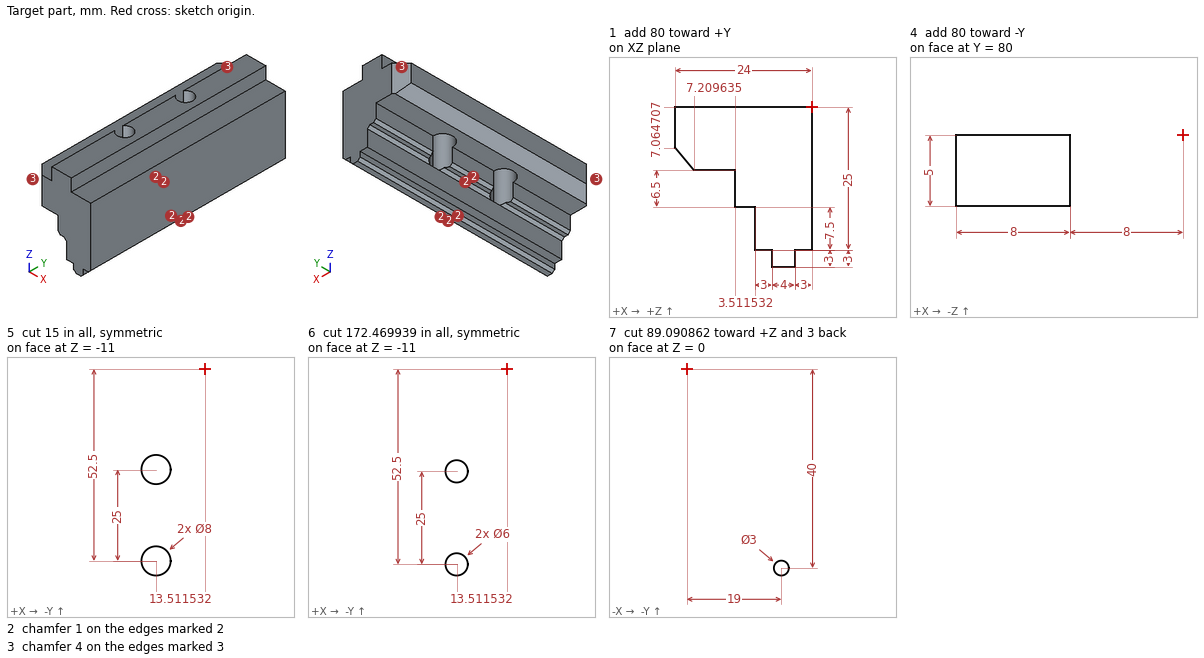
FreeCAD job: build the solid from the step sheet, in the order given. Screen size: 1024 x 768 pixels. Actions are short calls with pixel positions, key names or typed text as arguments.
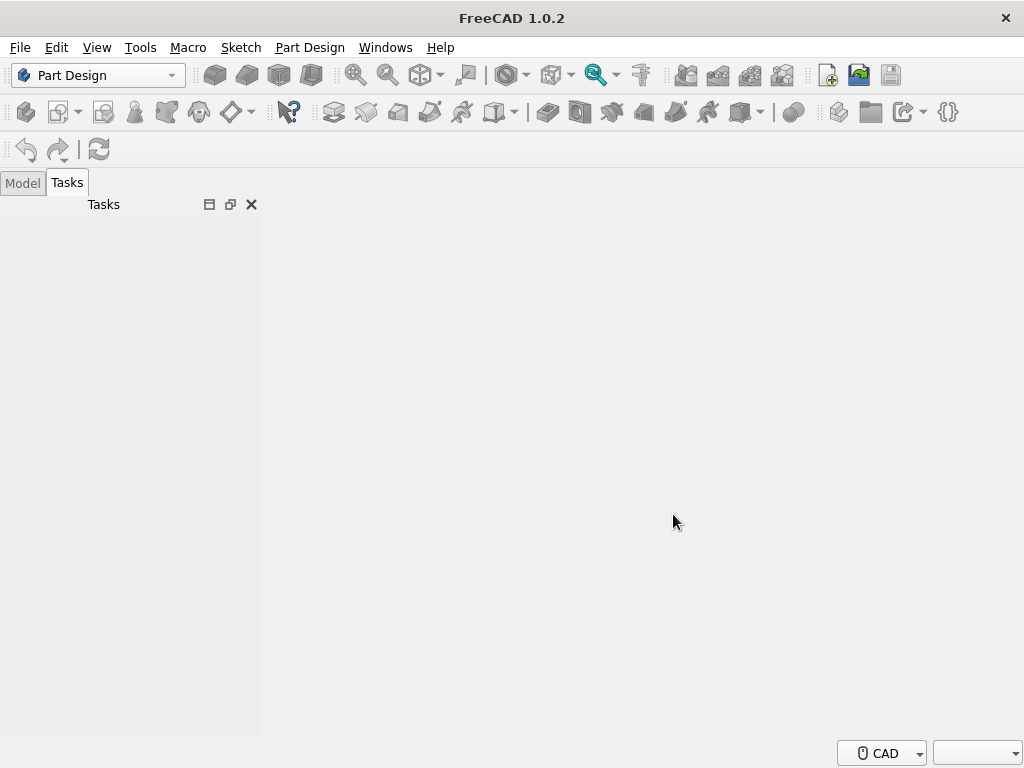
key(ctrl+n)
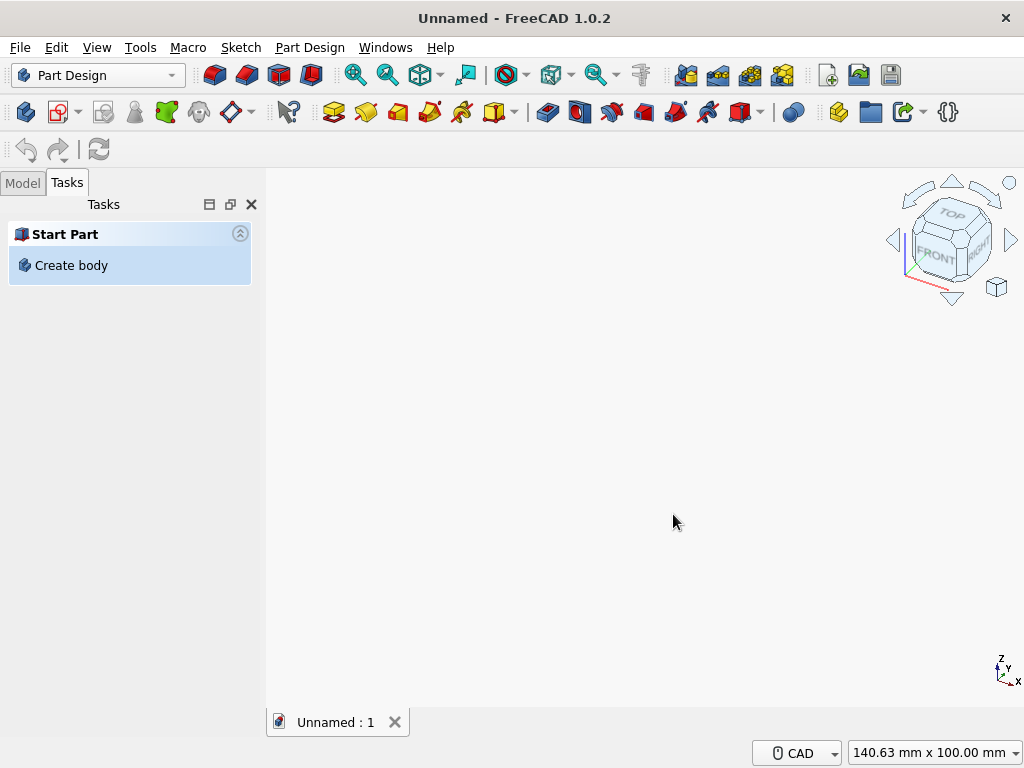
click(58, 112)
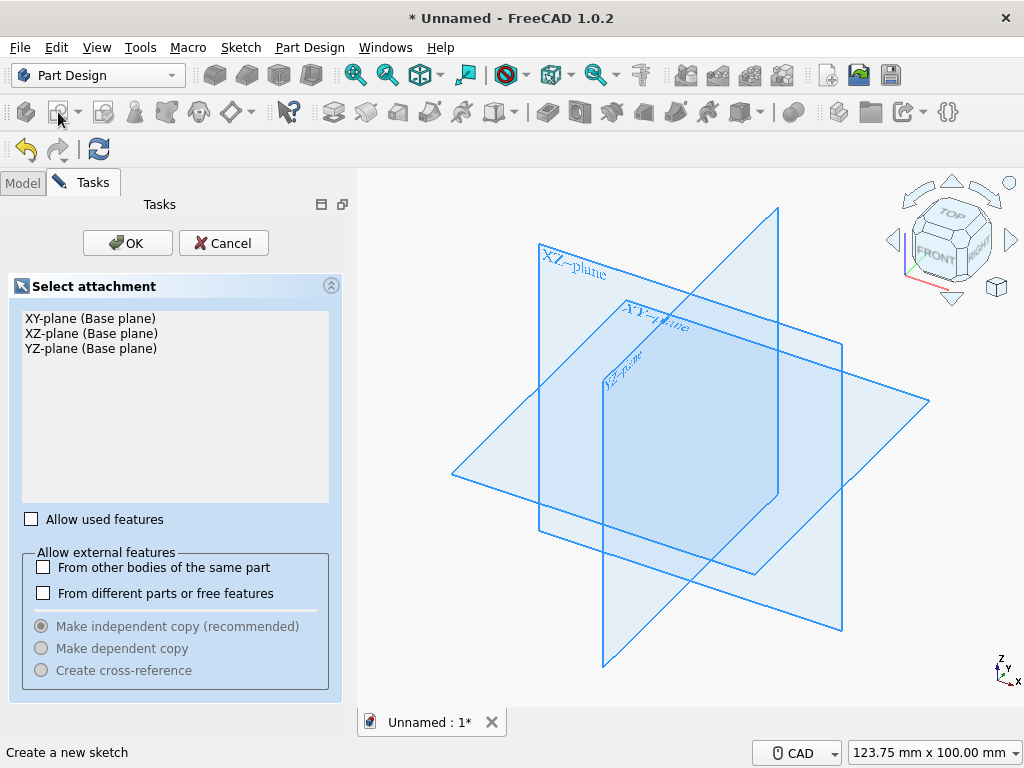
click(82, 334)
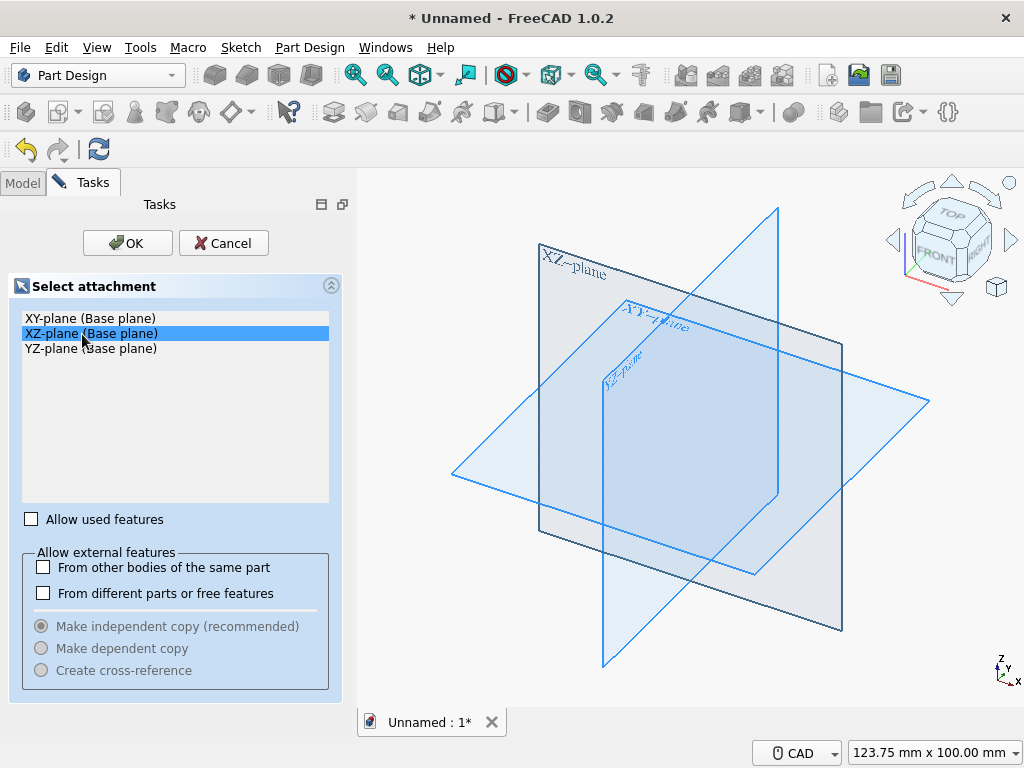
click(128, 243)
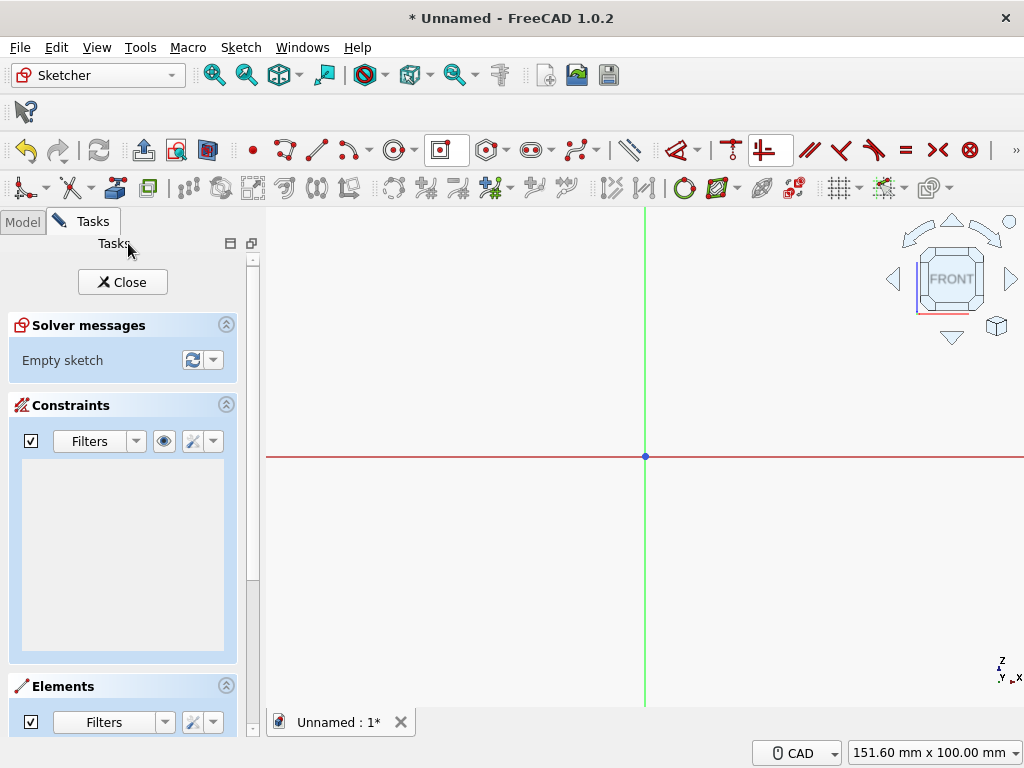
scroll(592, 584, up, 4)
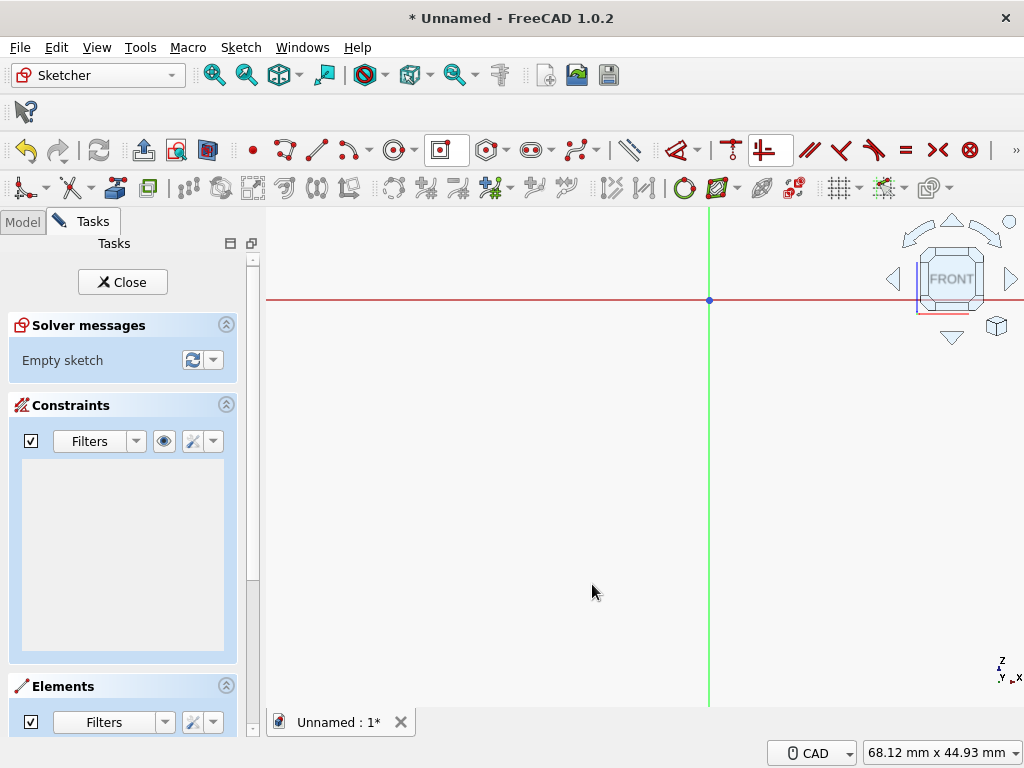
key(g)
key(m)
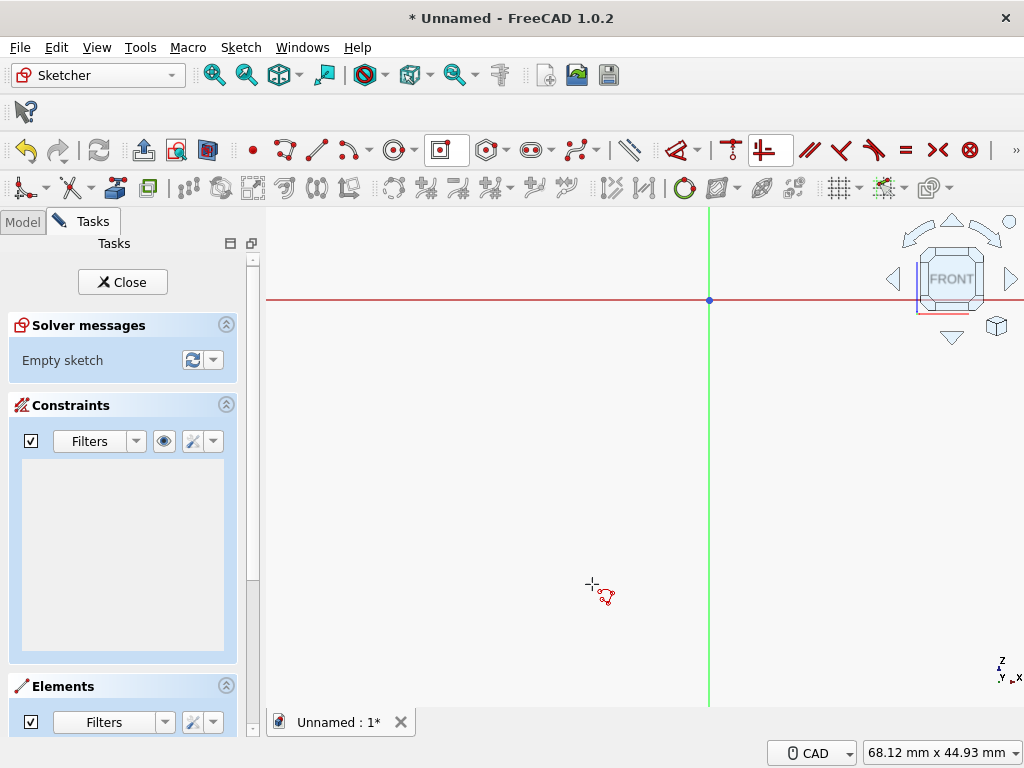
click(709, 300)
click(700, 579)
click(676, 579)
click(676, 612)
click(632, 612)
click(632, 579)
click(598, 579)
click(598, 495)
click(559, 495)
click(559, 423)
click(479, 423)
click(442, 379)
click(442, 309)
click(709, 300)
key(Escape)
key(Escape)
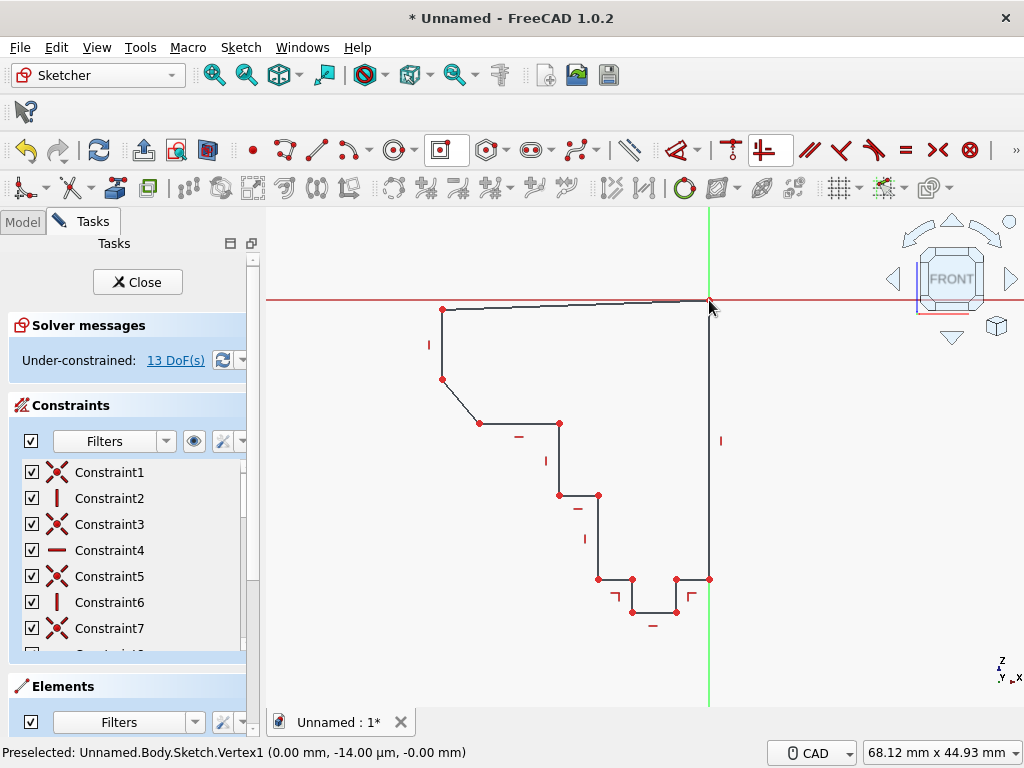
click(629, 303)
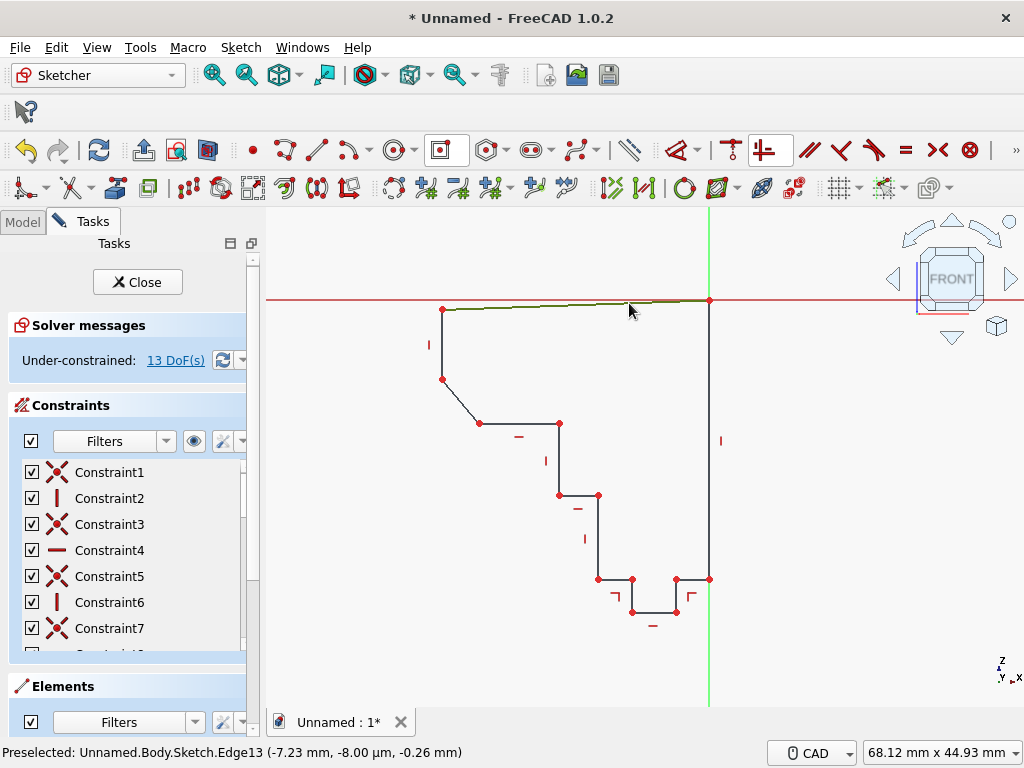
key(h)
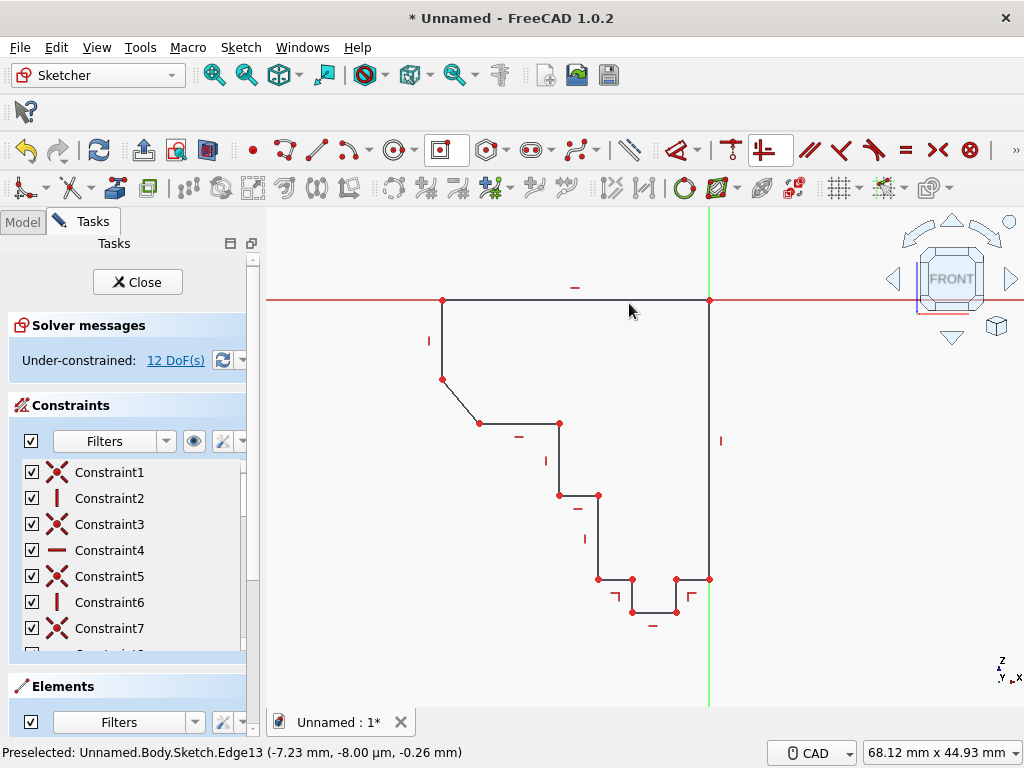
scroll(699, 580, up, 2)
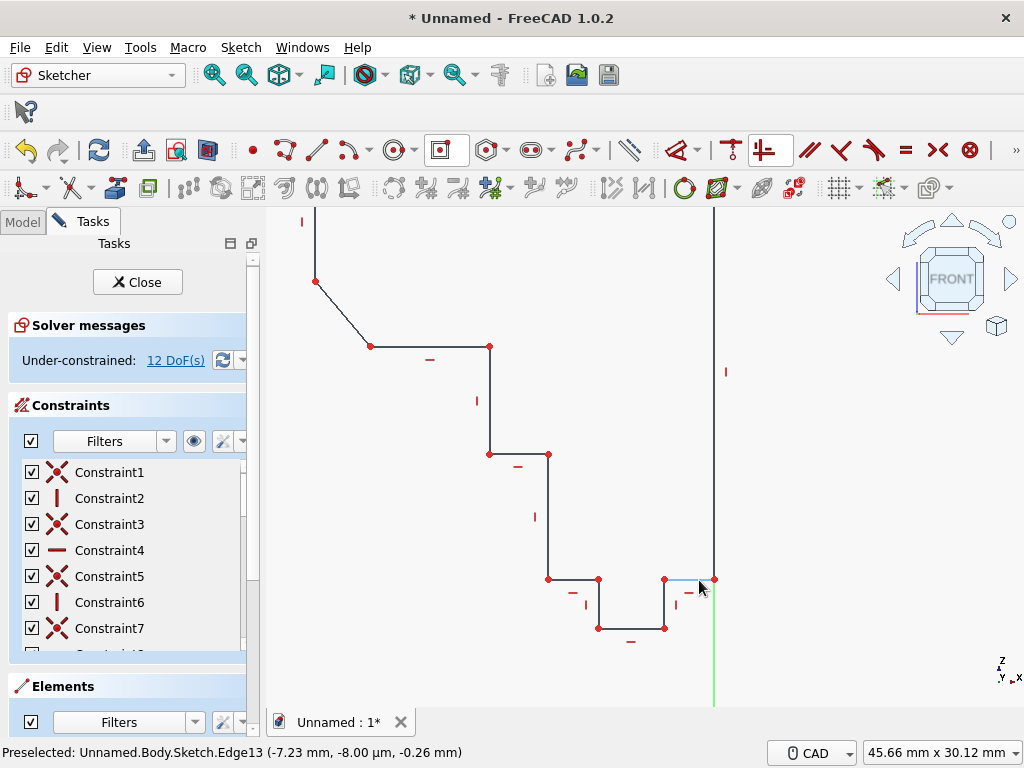
click(699, 580)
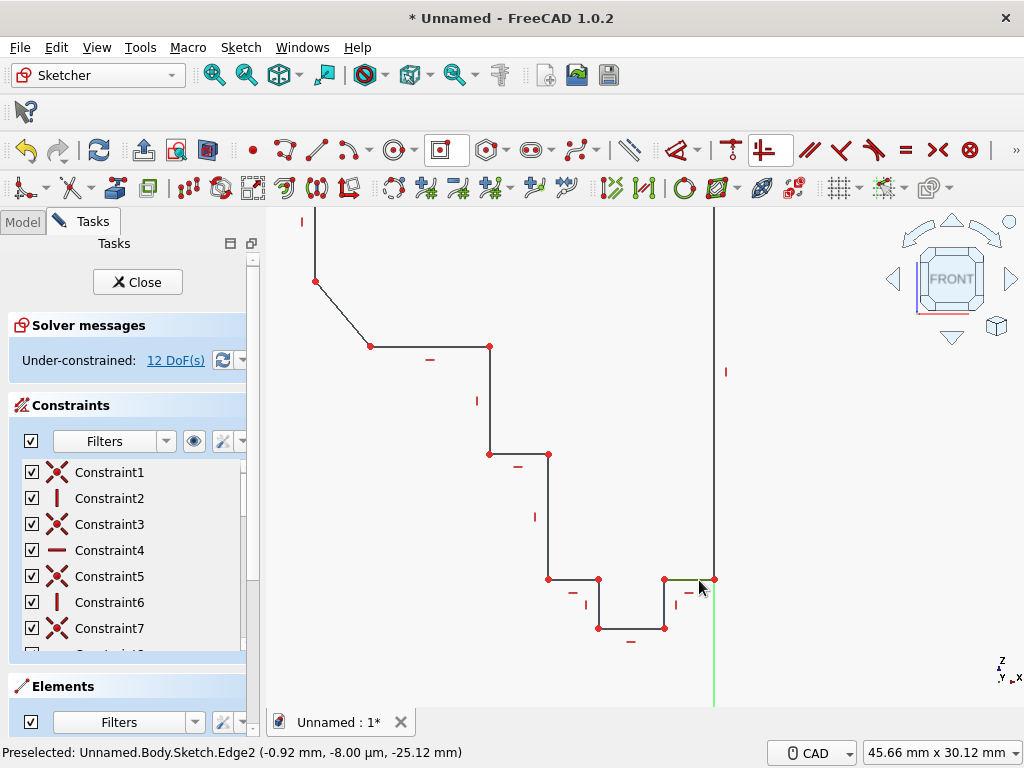
key(l)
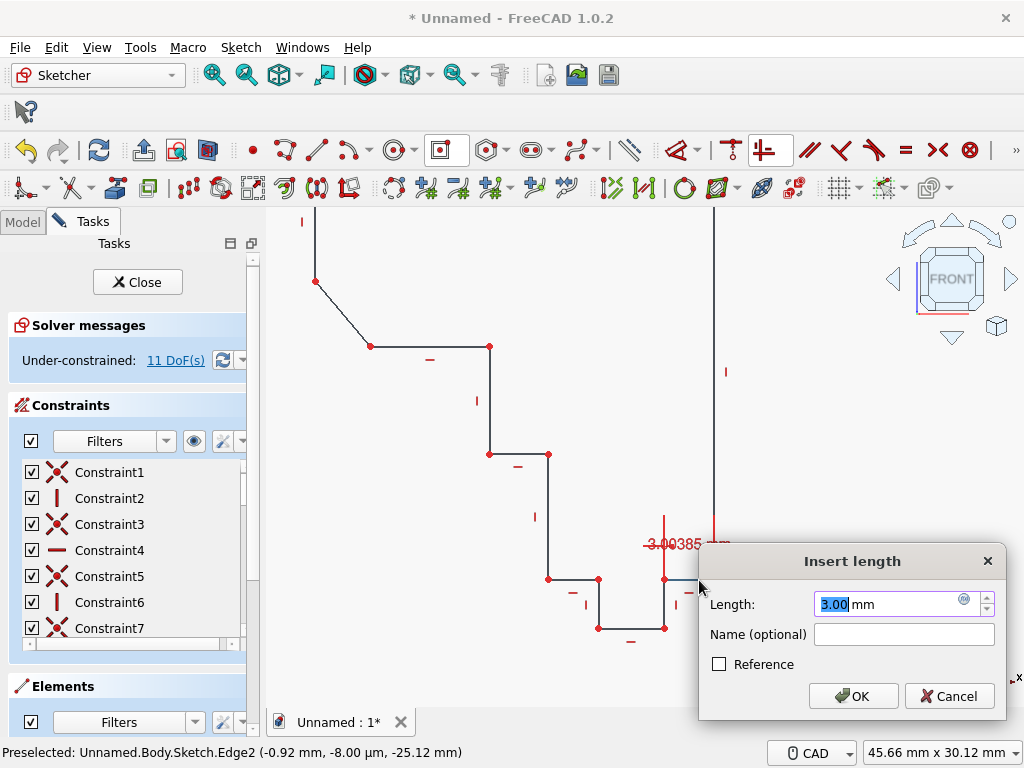
text(3)
key(Return)